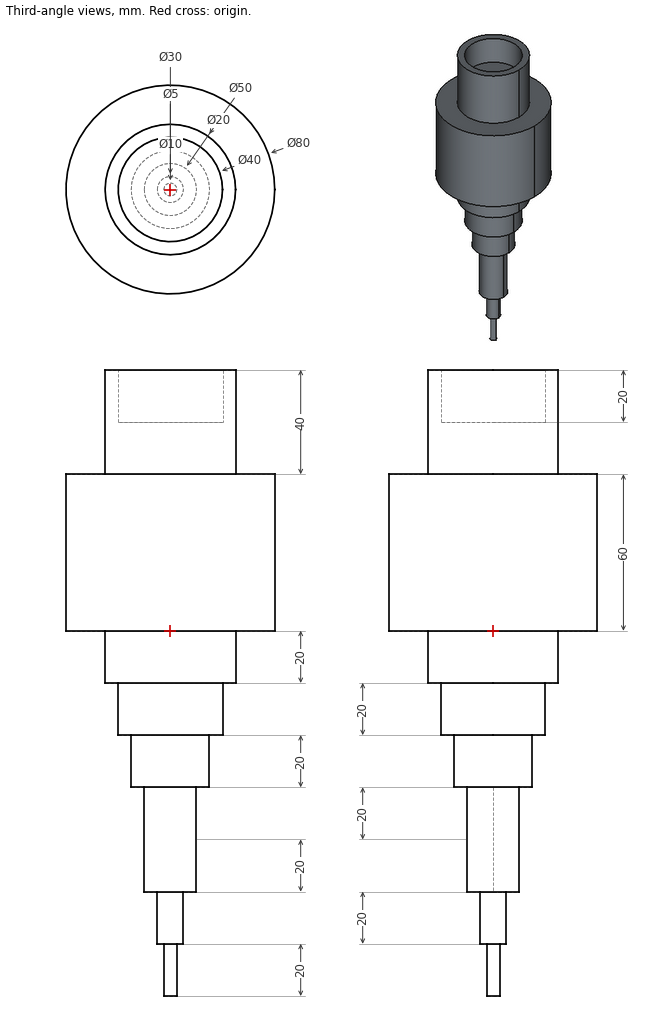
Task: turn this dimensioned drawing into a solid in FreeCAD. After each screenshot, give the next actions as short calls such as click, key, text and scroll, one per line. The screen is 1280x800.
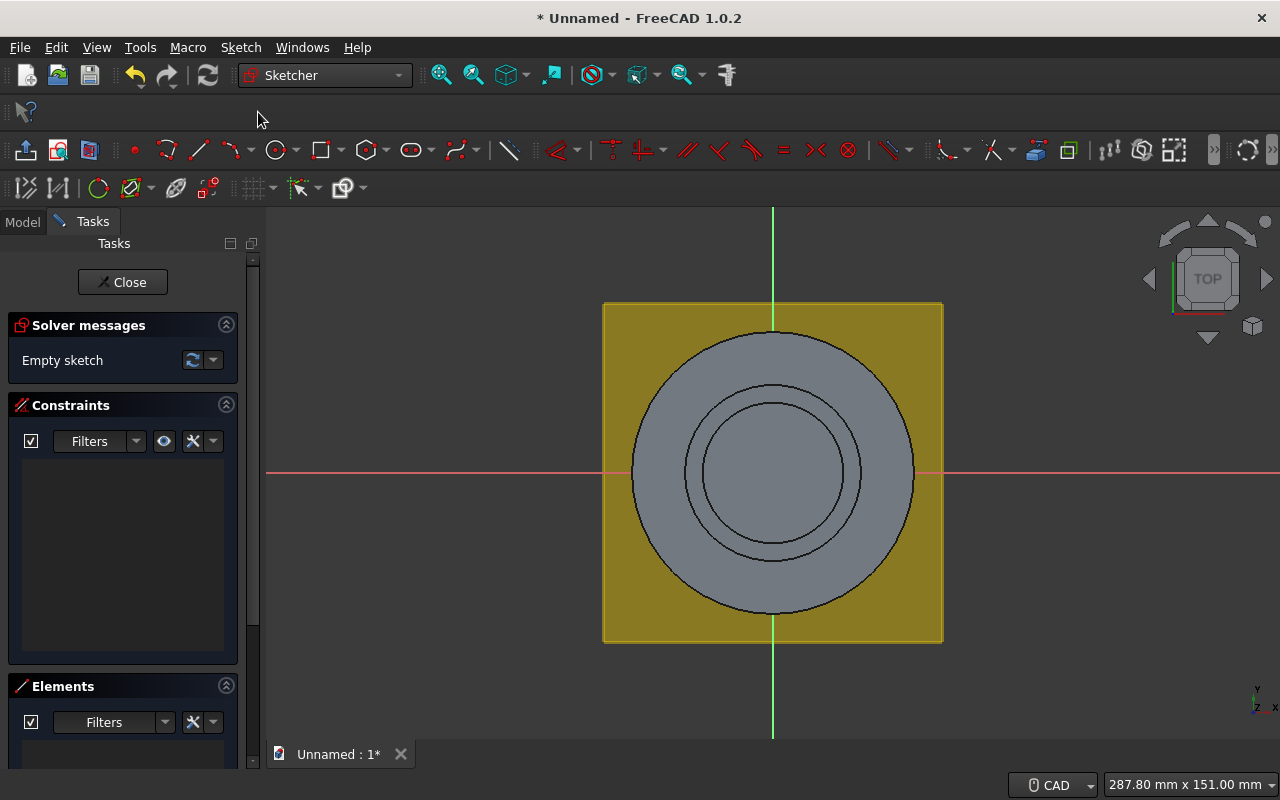
click(90, 150)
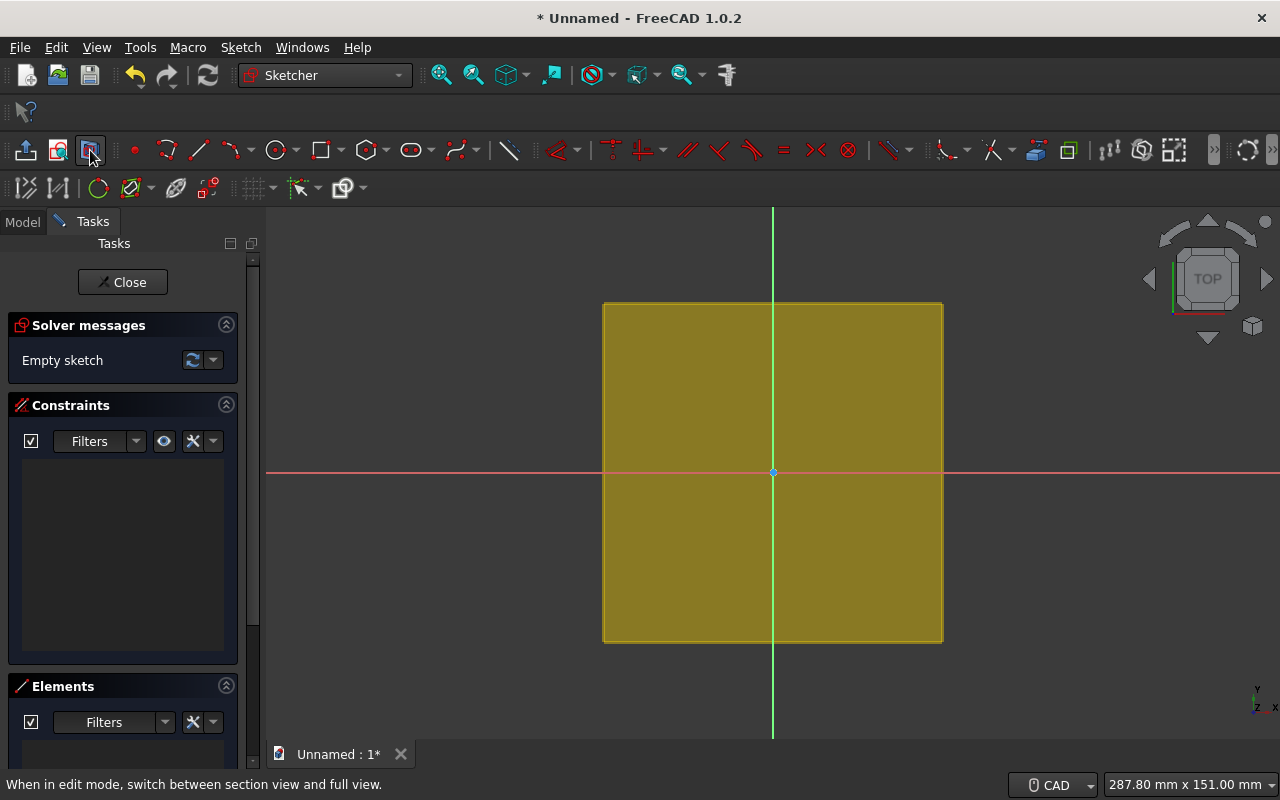
scroll(856, 473, up, 3)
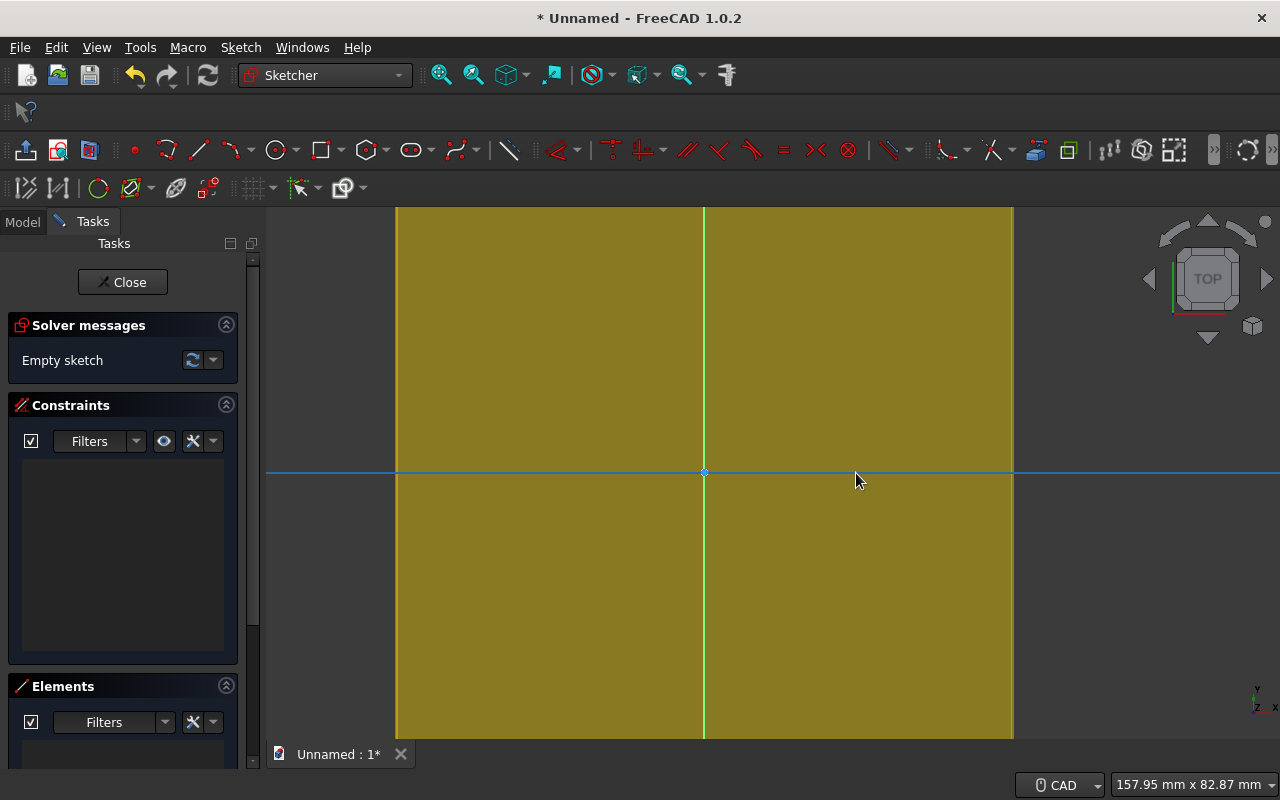
click(276, 150)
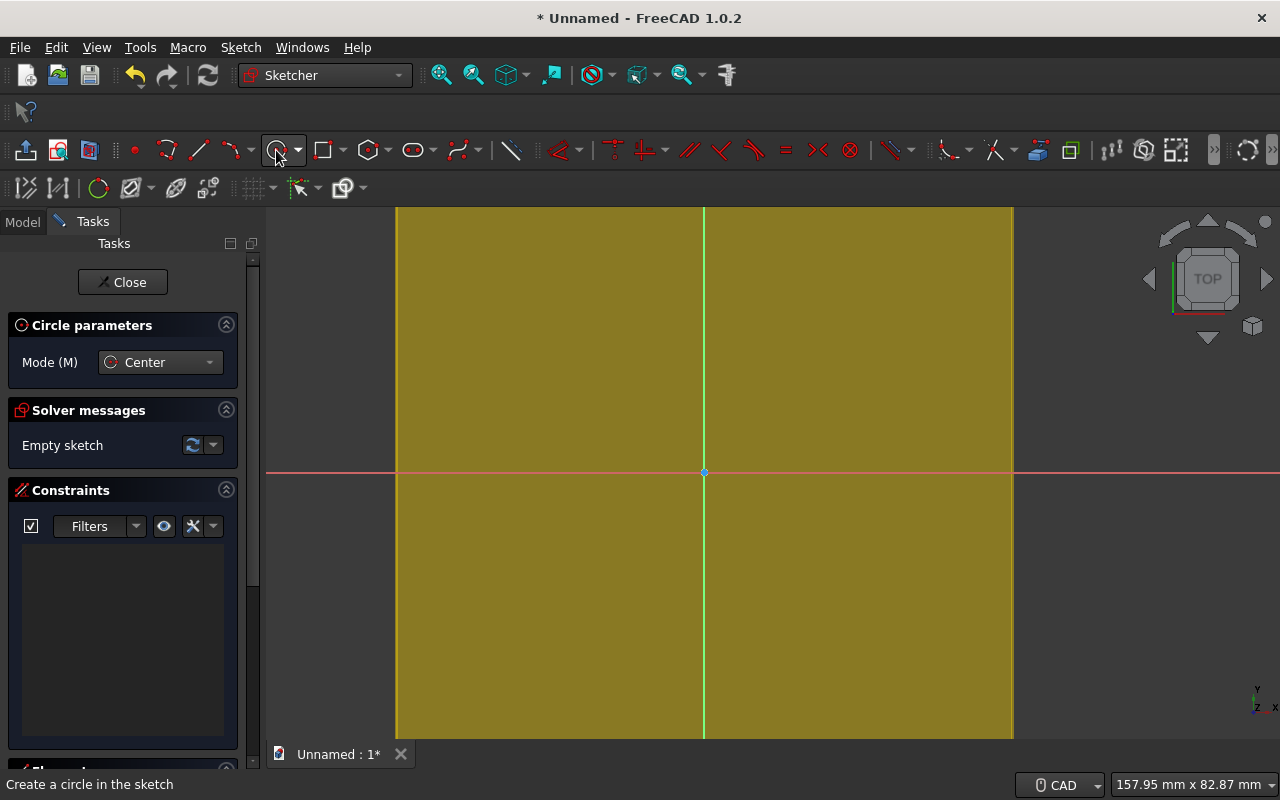
click(704, 473)
click(818, 359)
key(Escape)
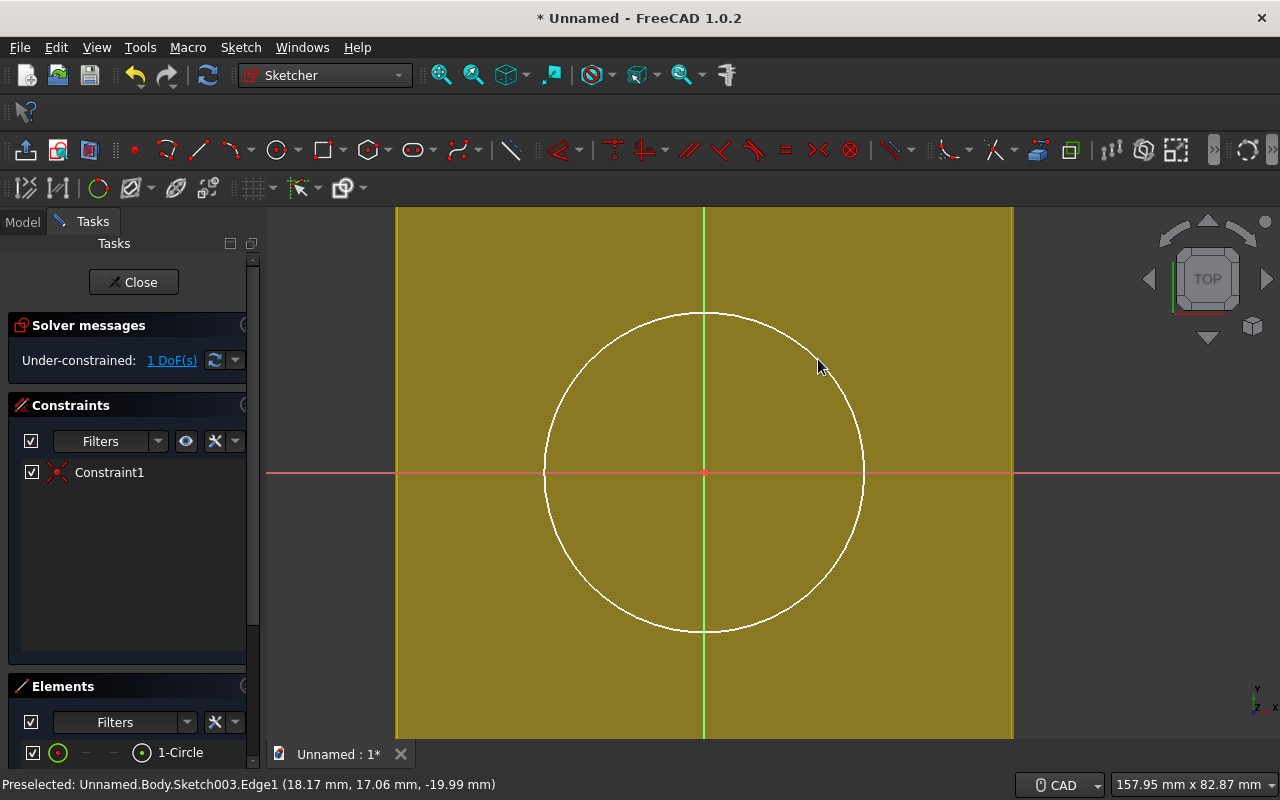
click(558, 150)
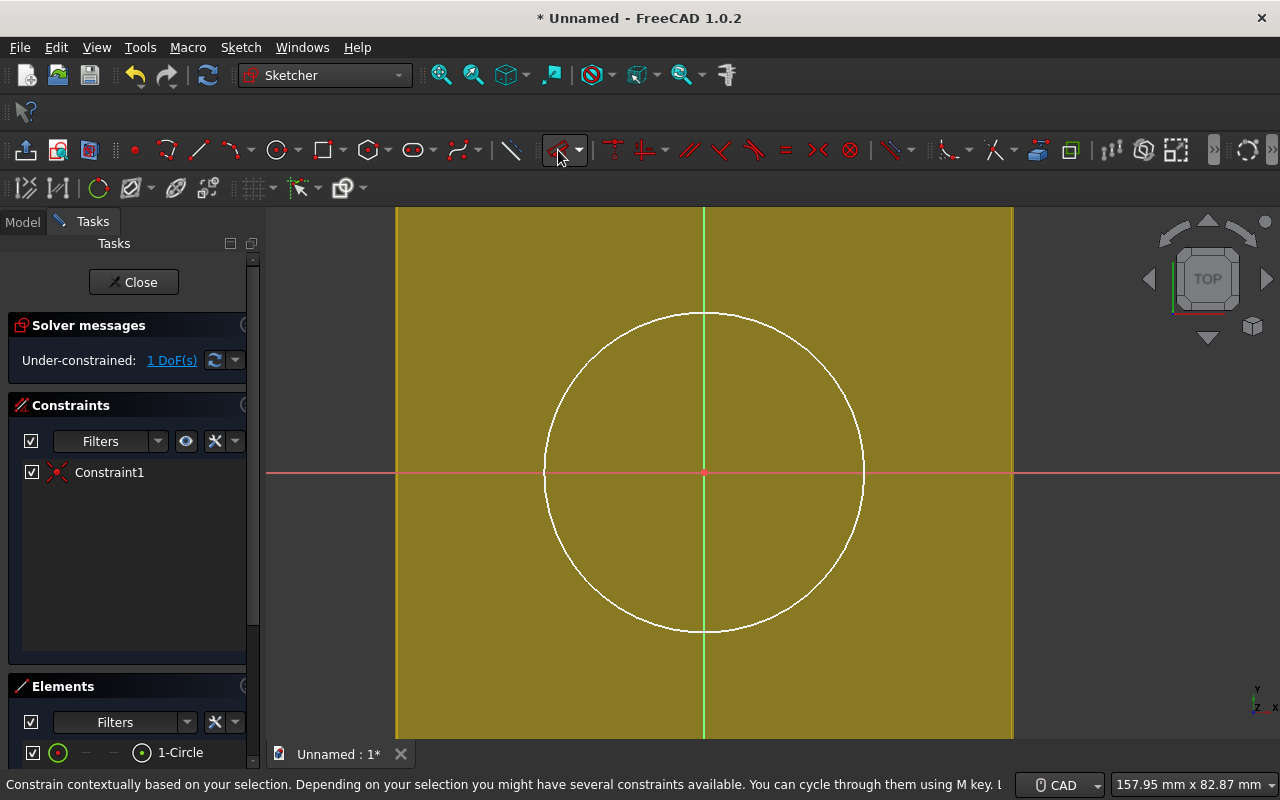
click(817, 359)
click(840, 336)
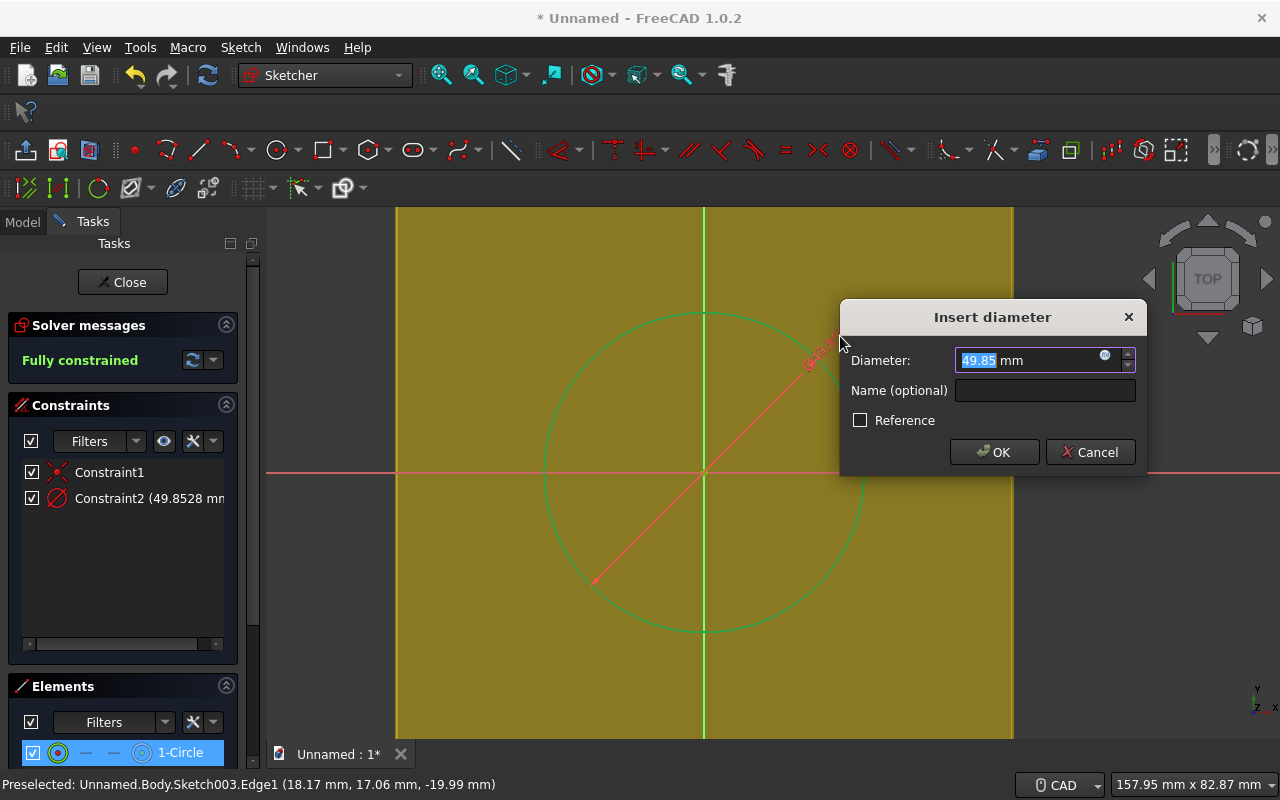
text(50)
key(Return)
key(Escape)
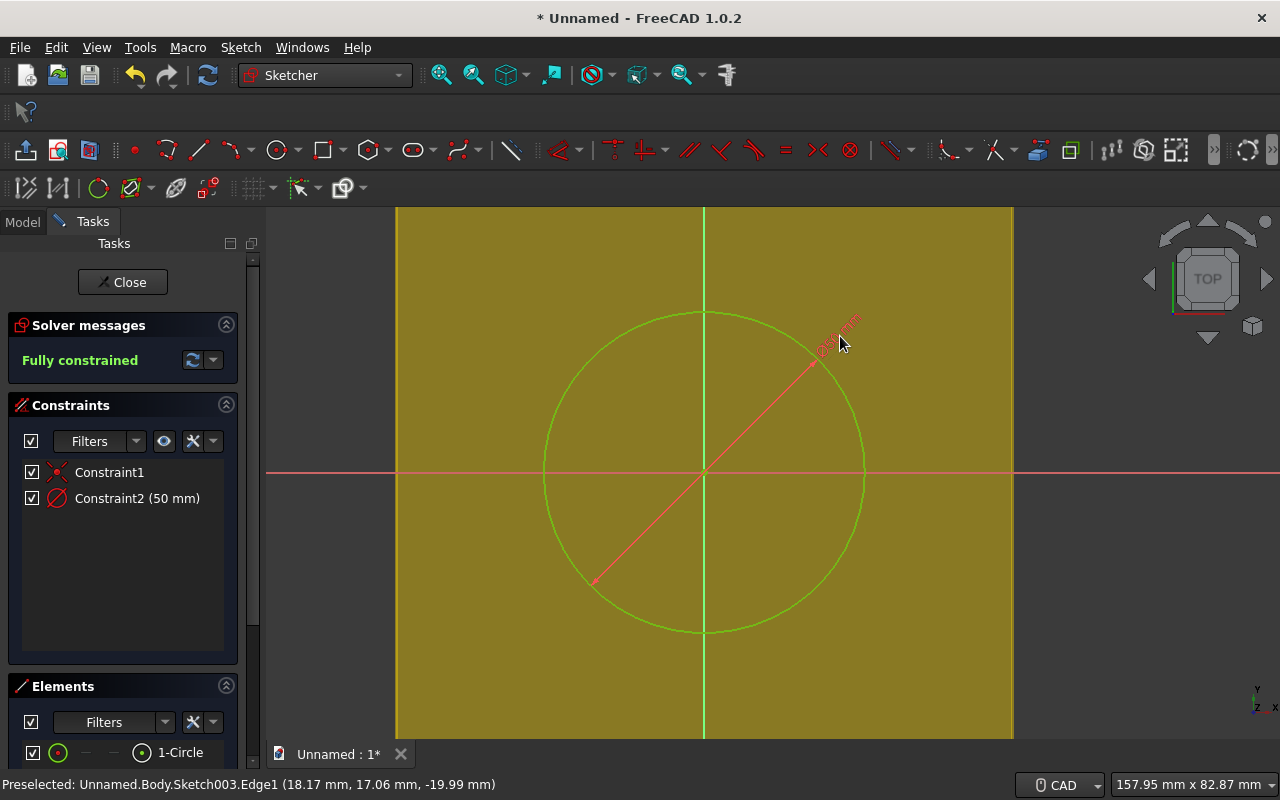
click(123, 282)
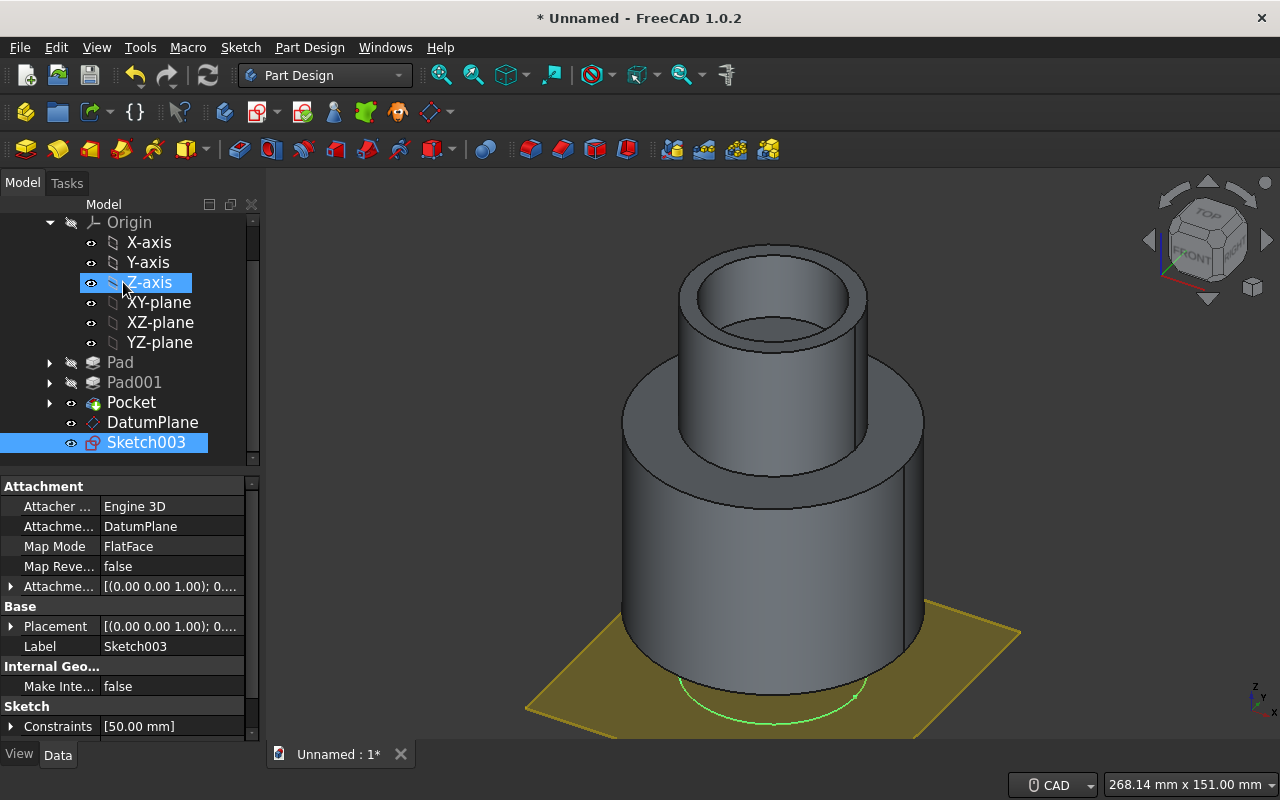
click(26, 150)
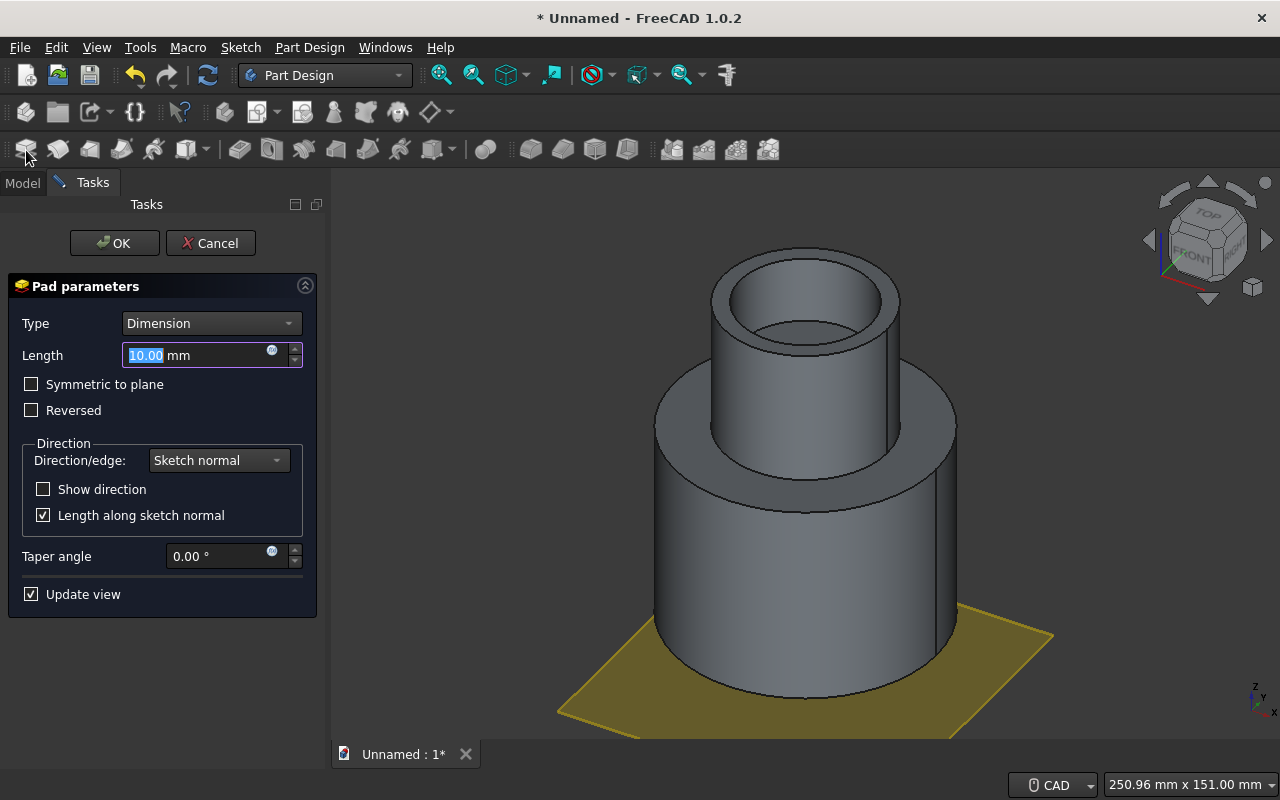
text(20)
key(Tab)